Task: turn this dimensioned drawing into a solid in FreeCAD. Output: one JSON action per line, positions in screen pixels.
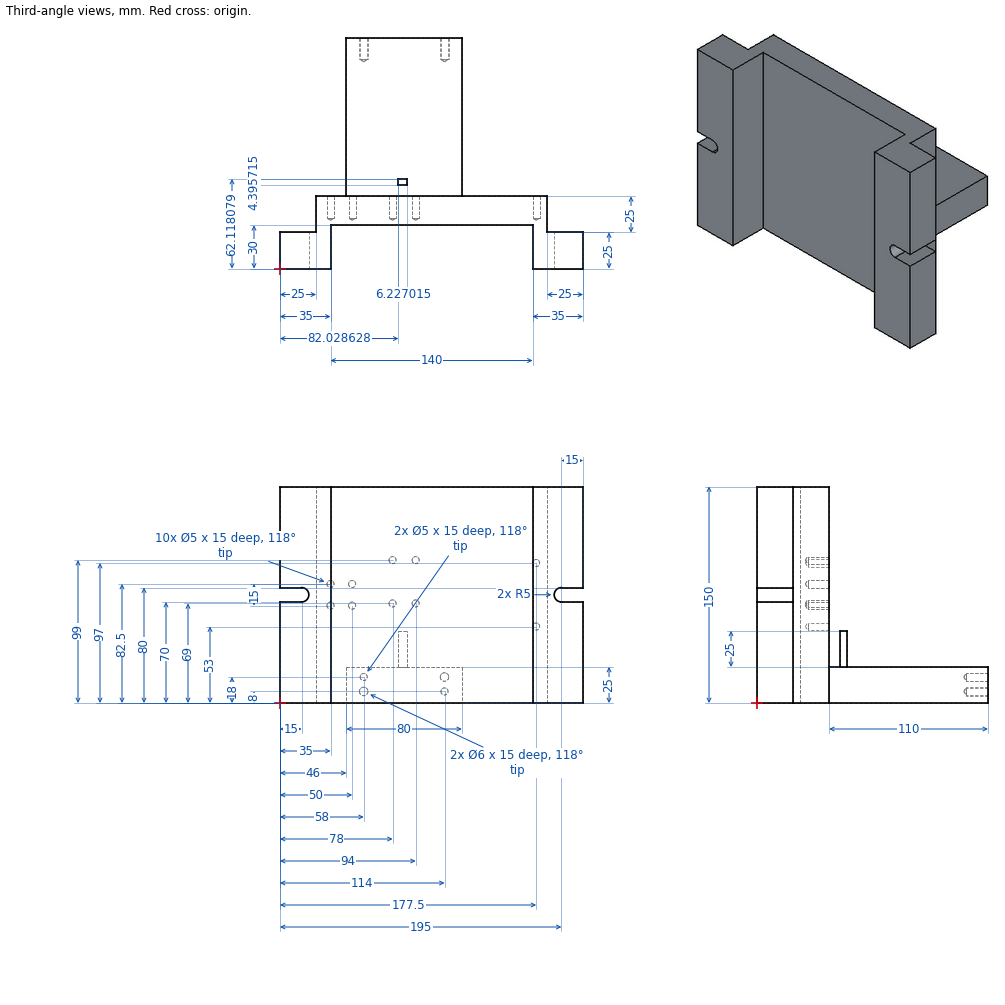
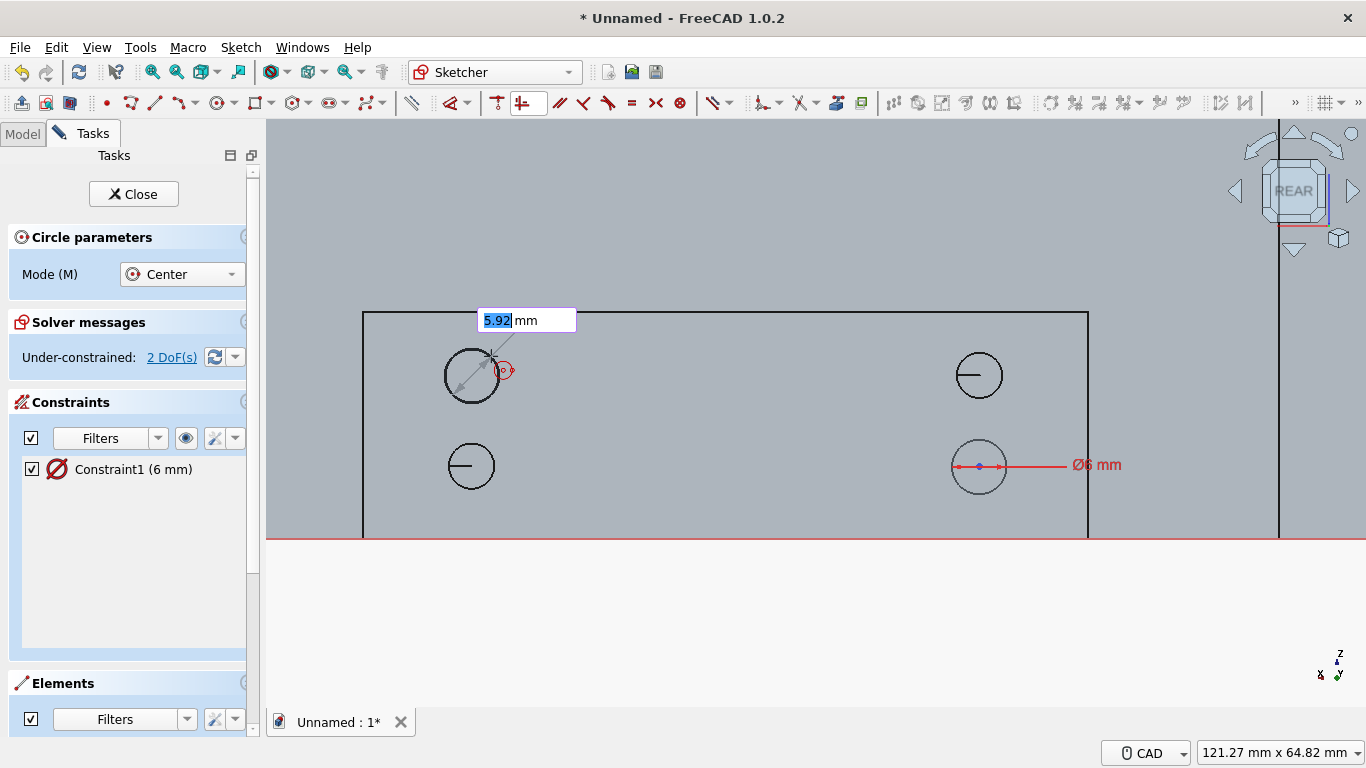
{"action": "type", "text": "6"}
{"action": "key", "text": "Return"}
{"action": "key", "text": "Escape"}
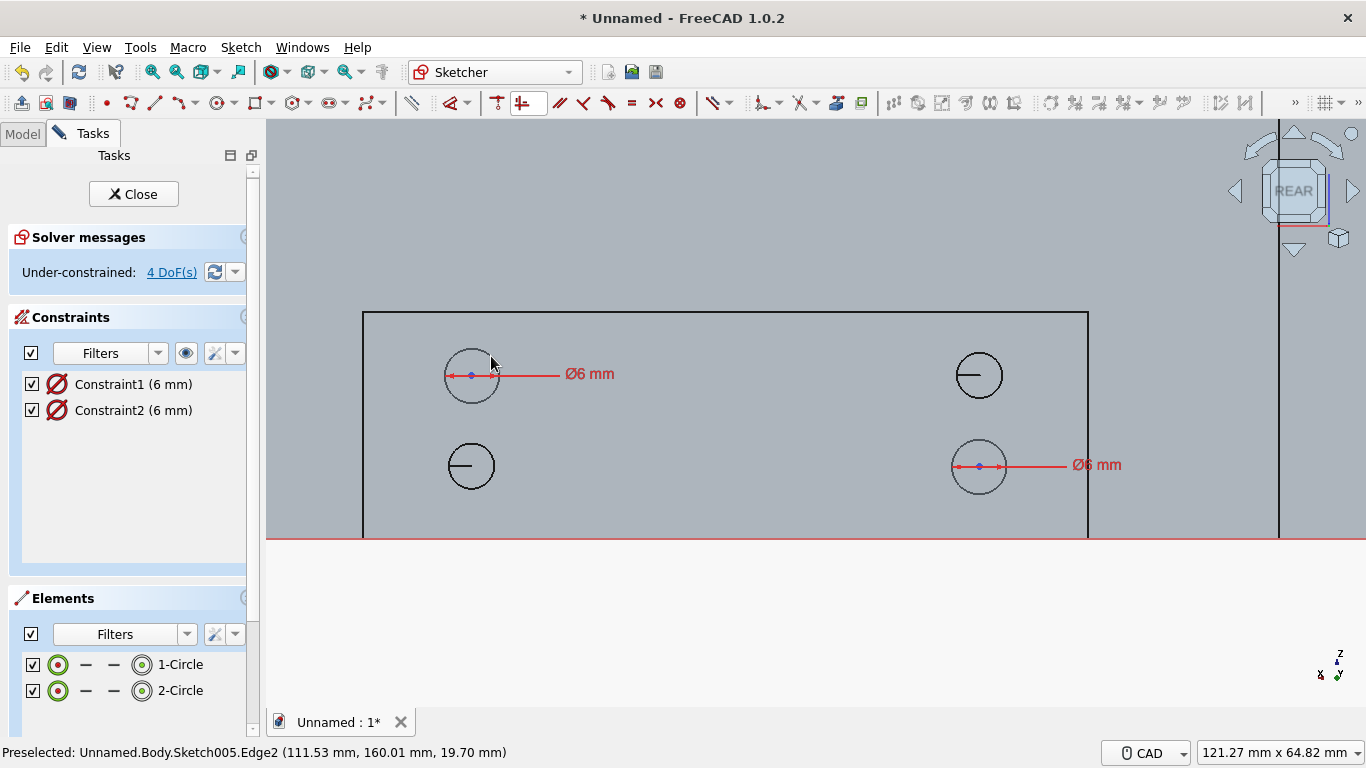
{"action": "key", "text": "d"}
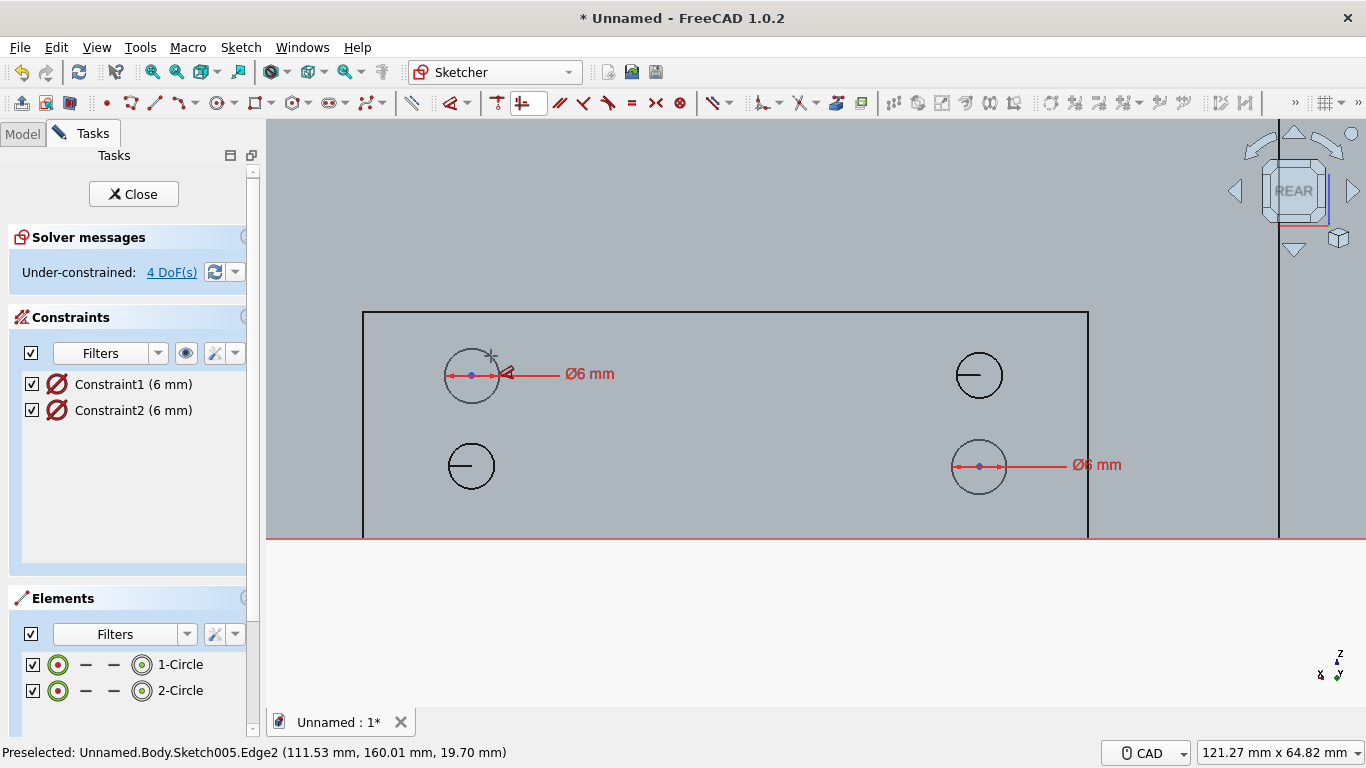
{"action": "left_click", "coordinate": [979, 467]}
{"action": "left_click", "coordinate": [945, 503]}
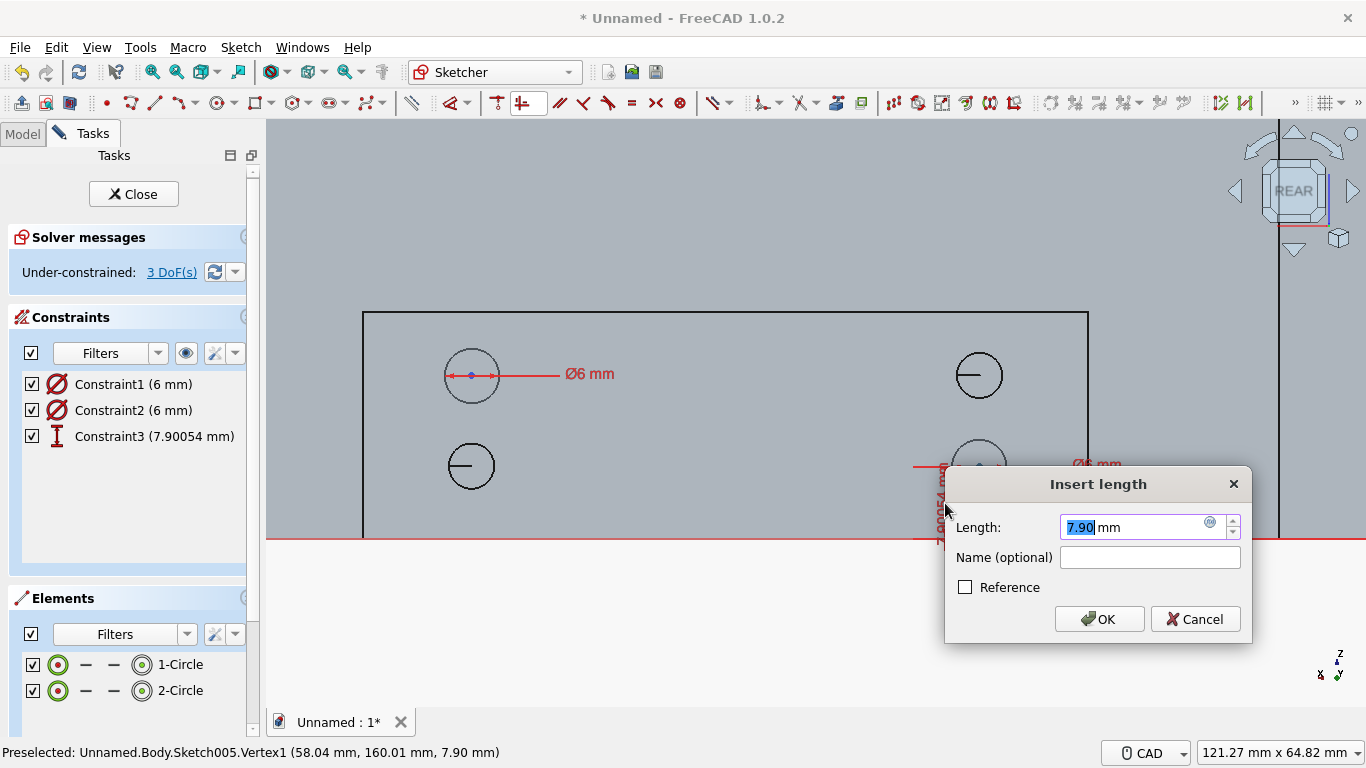
{"action": "type", "text": "8"}
{"action": "key", "text": "Return"}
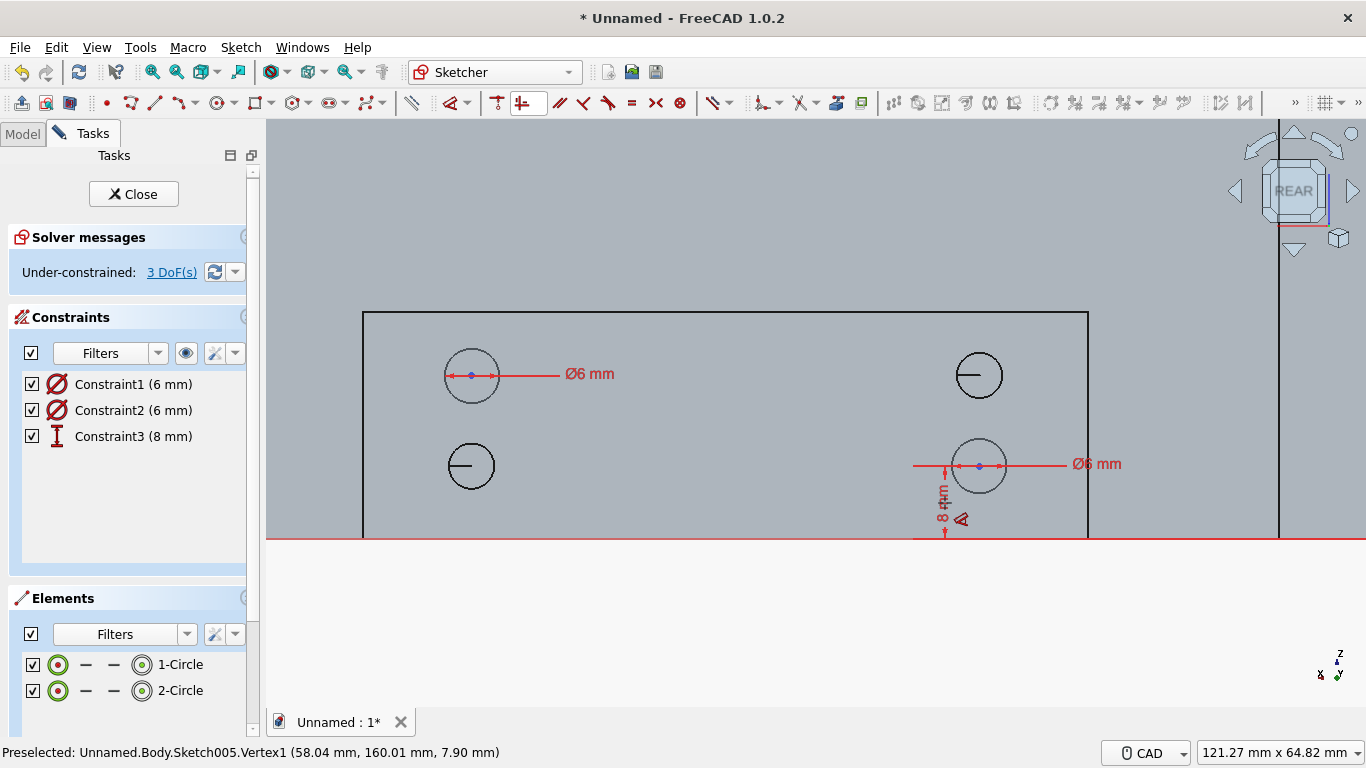
{"action": "left_click", "coordinate": [979, 466]}
{"action": "left_click", "coordinate": [1090, 573]}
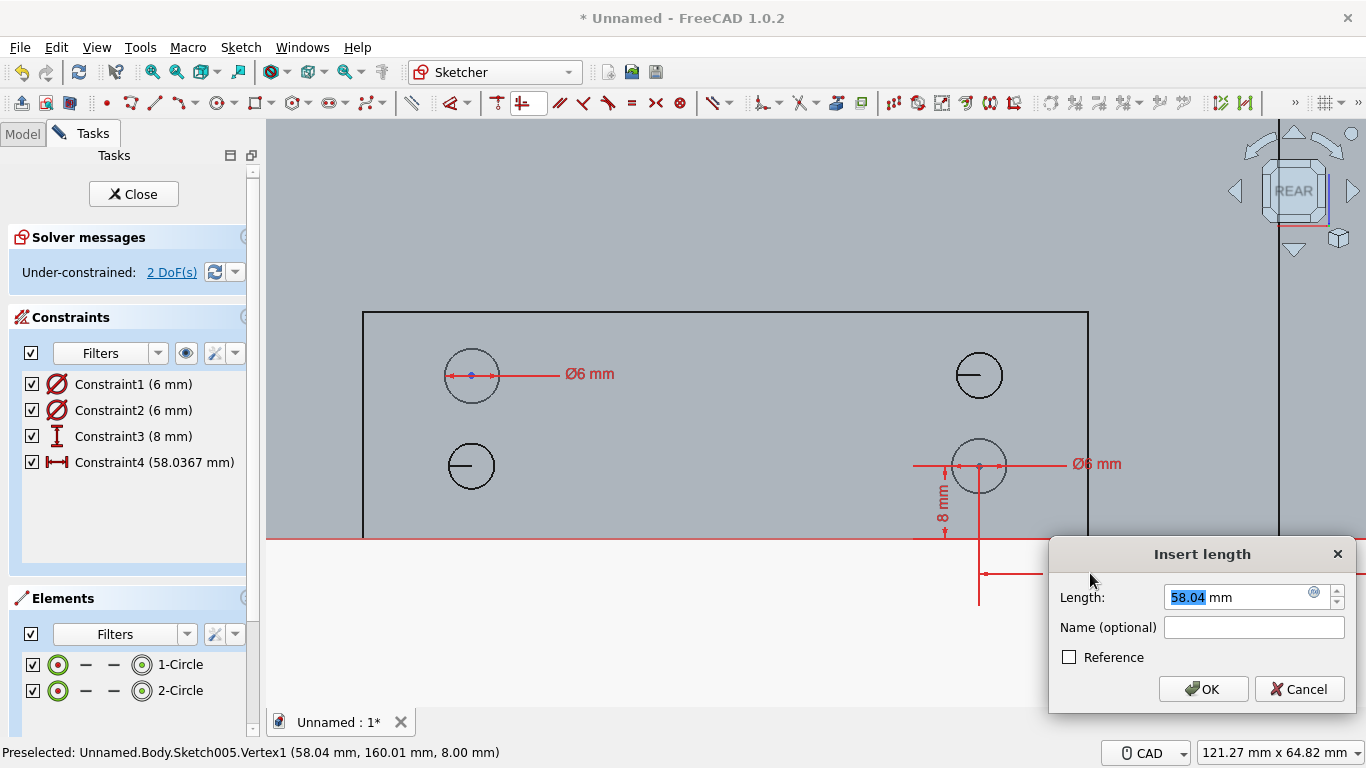
{"action": "type", "text": "58"}
{"action": "key", "text": "Return"}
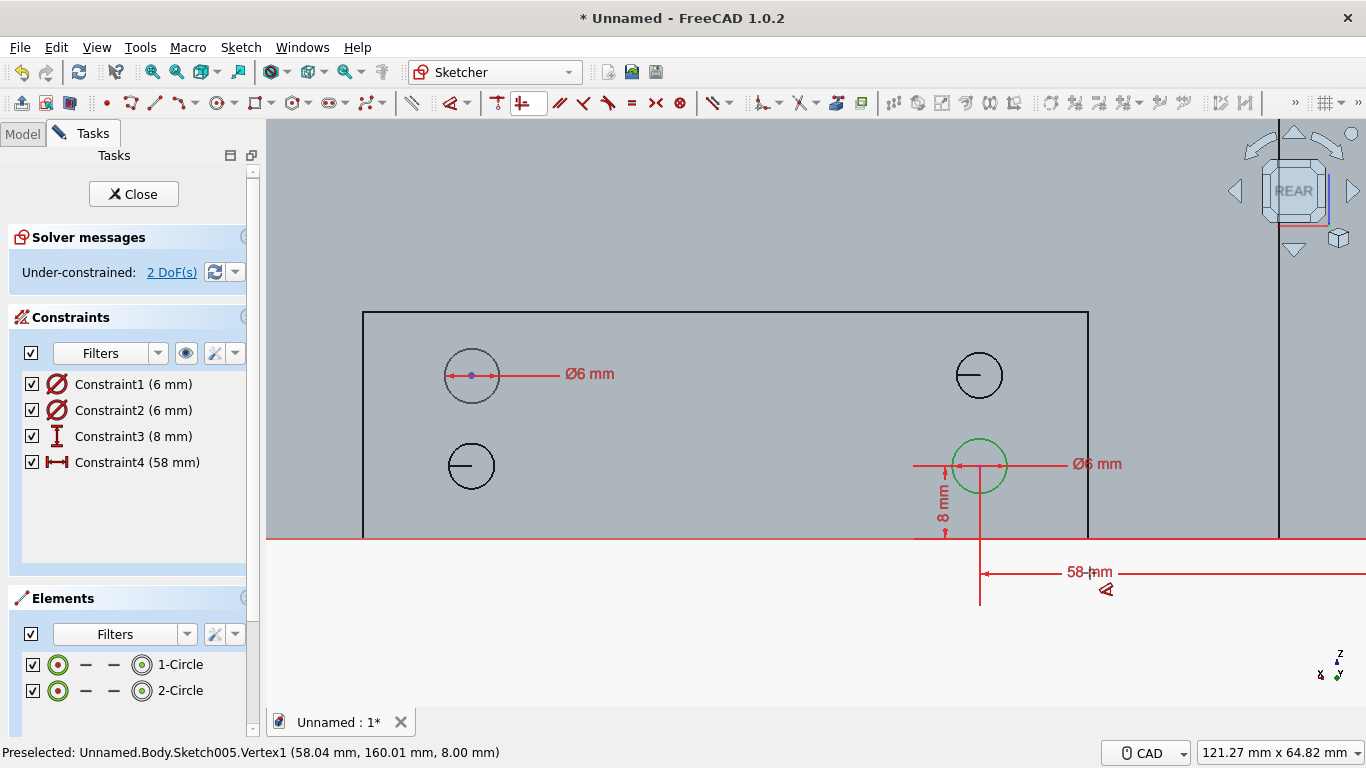
{"action": "left_click", "coordinate": [472, 376]}
{"action": "left_click", "coordinate": [438, 457]}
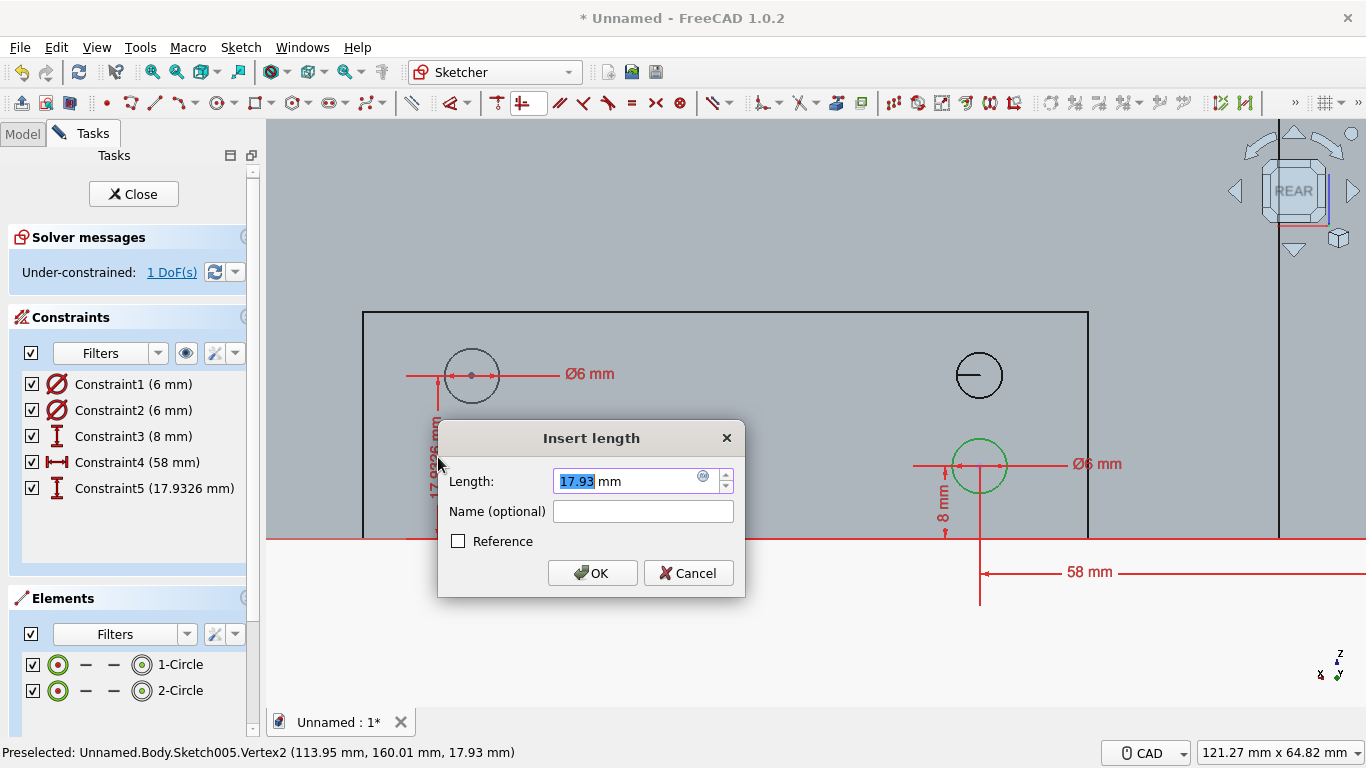
{"action": "type", "text": "18"}
{"action": "key", "text": "Return"}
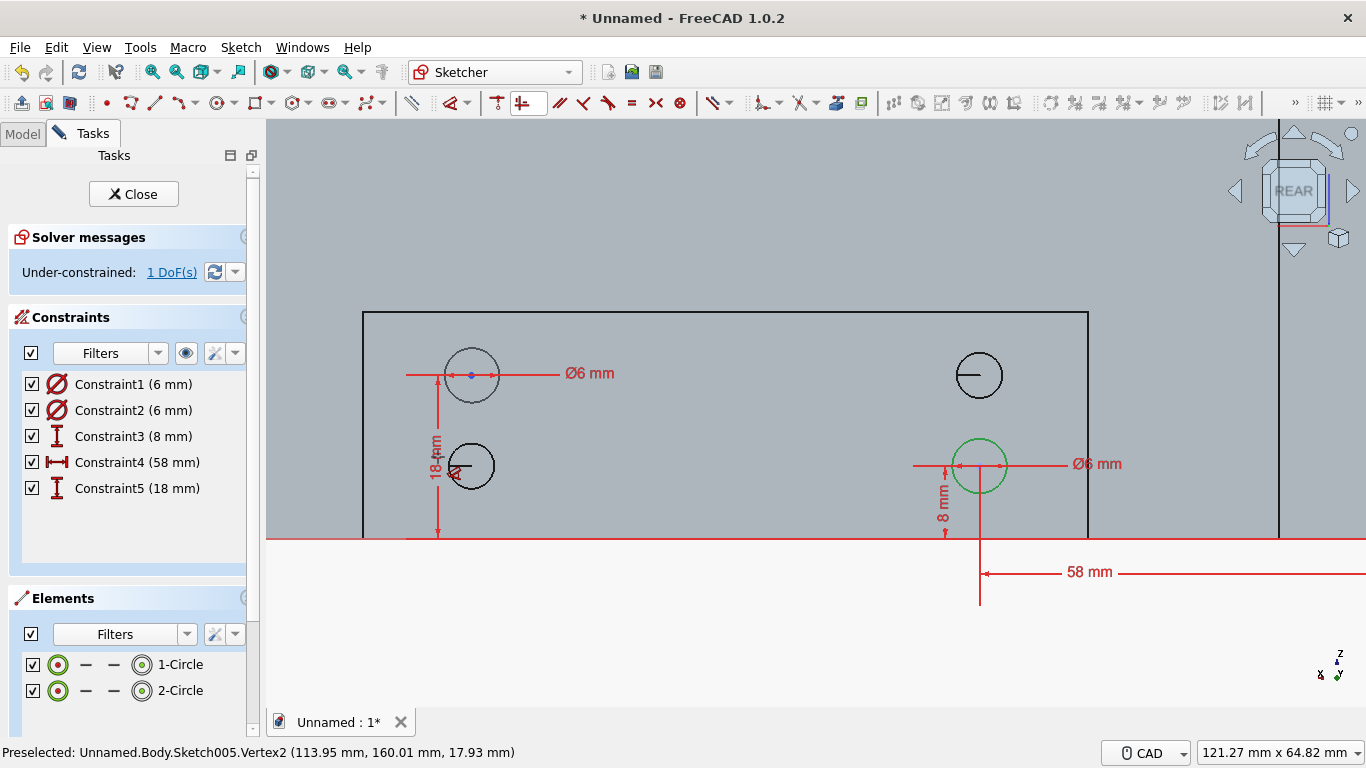
{"action": "left_click", "coordinate": [472, 375]}
{"action": "left_click", "coordinate": [837, 573]}